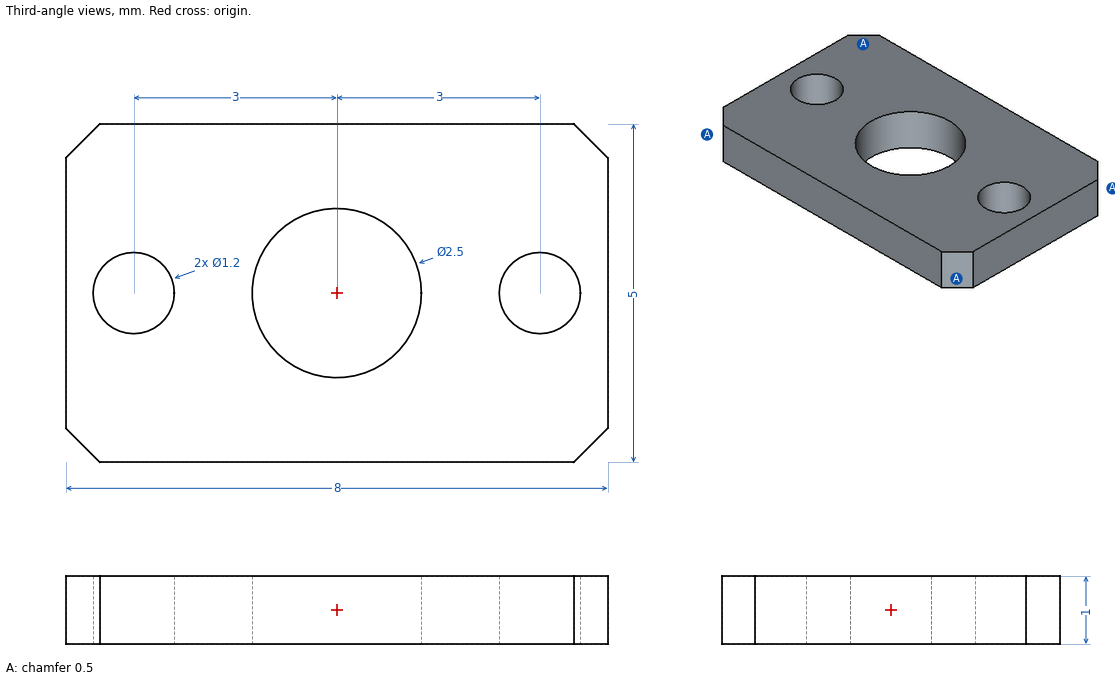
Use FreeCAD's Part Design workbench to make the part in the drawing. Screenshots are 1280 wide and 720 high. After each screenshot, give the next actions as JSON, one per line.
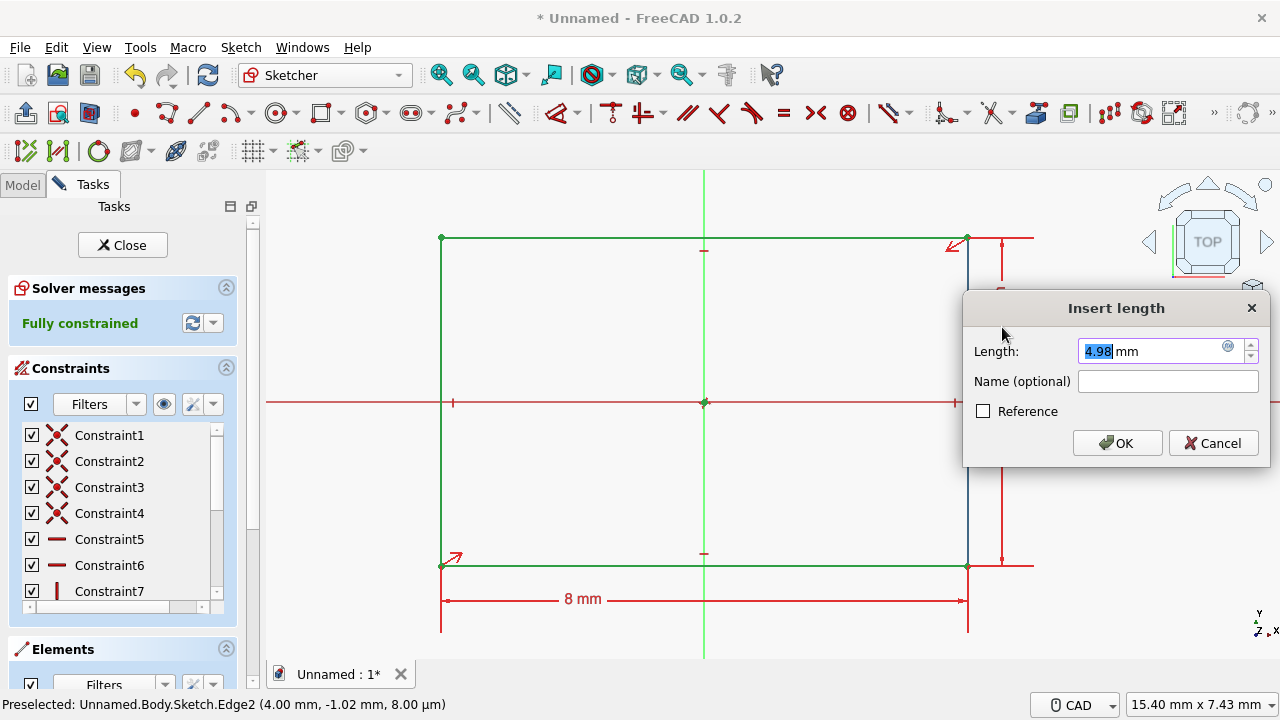
{"action": "type", "text": "5"}
{"action": "key", "text": "Return"}
{"action": "key", "text": "Escape"}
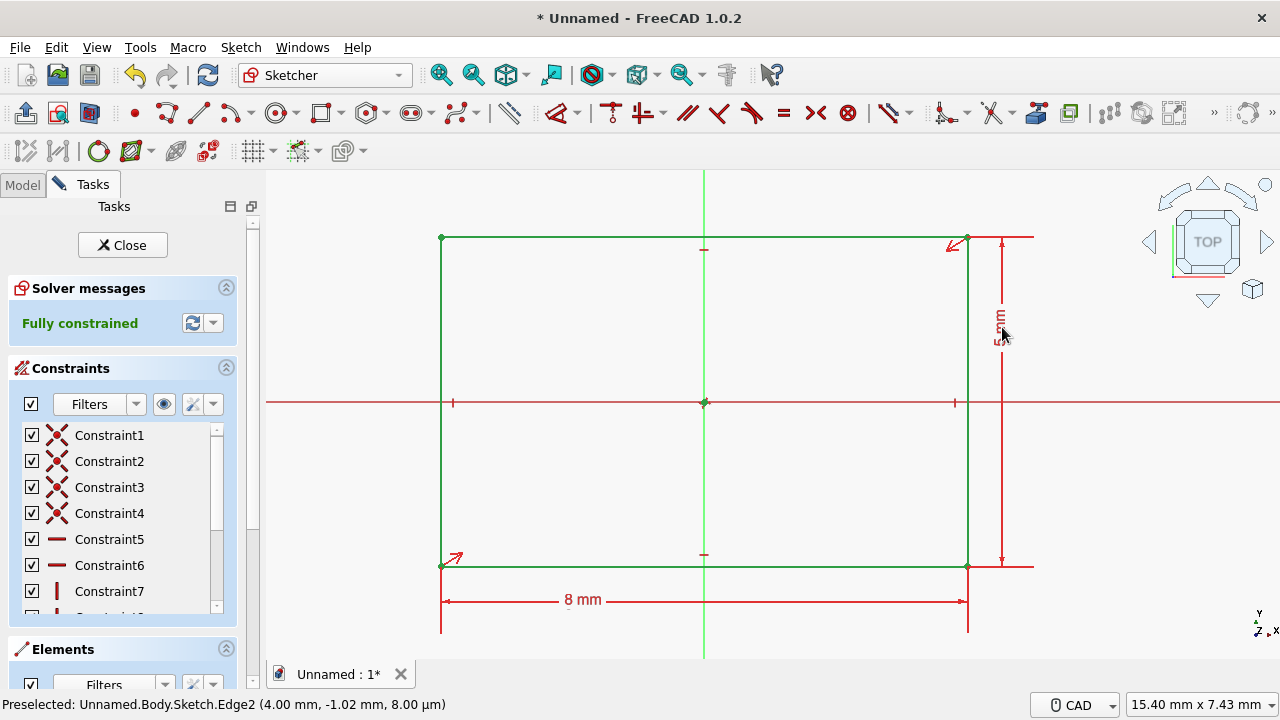
{"action": "left_click", "coordinate": [123, 245]}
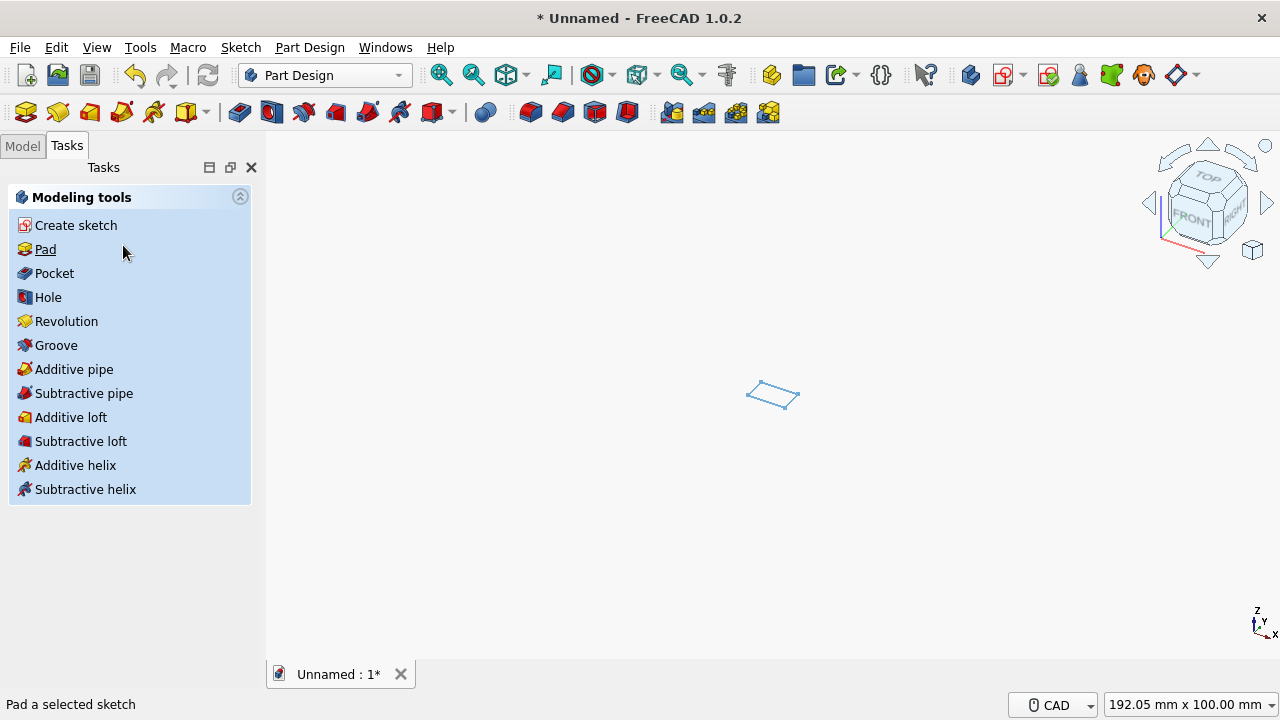
{"action": "left_click", "coordinate": [26, 112]}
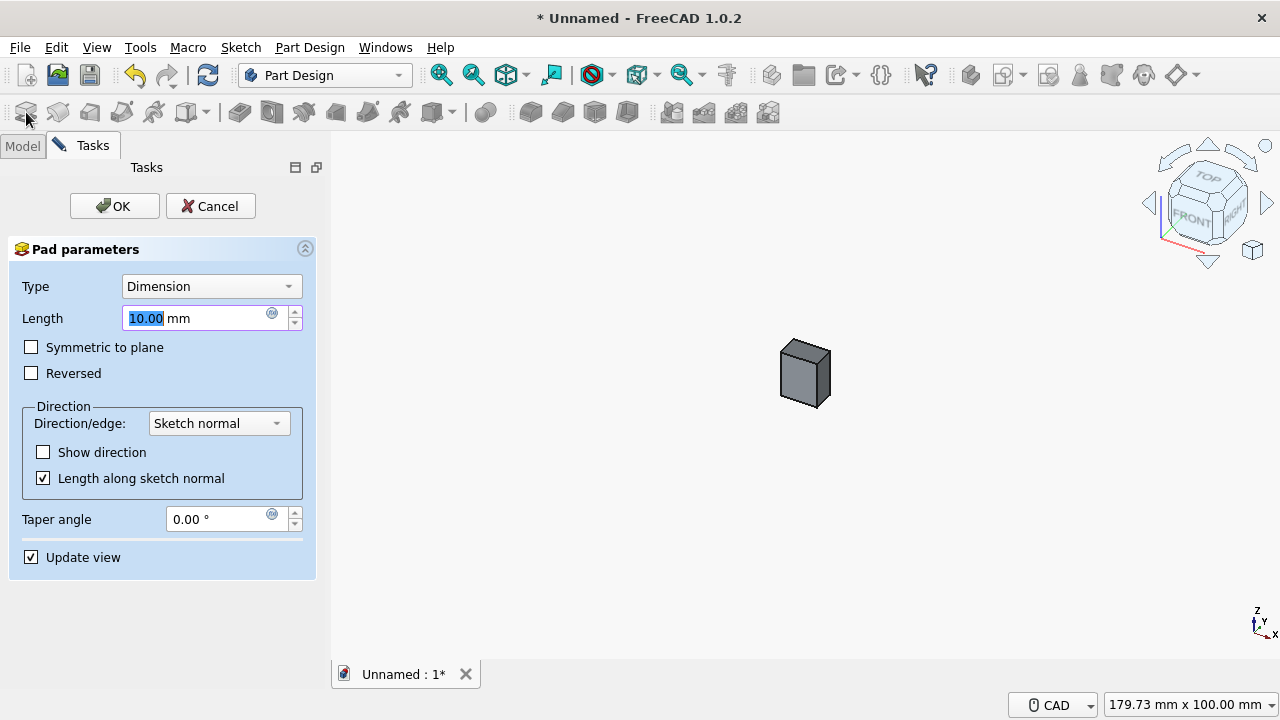
{"action": "type", "text": "1"}
{"action": "key", "text": "Tab"}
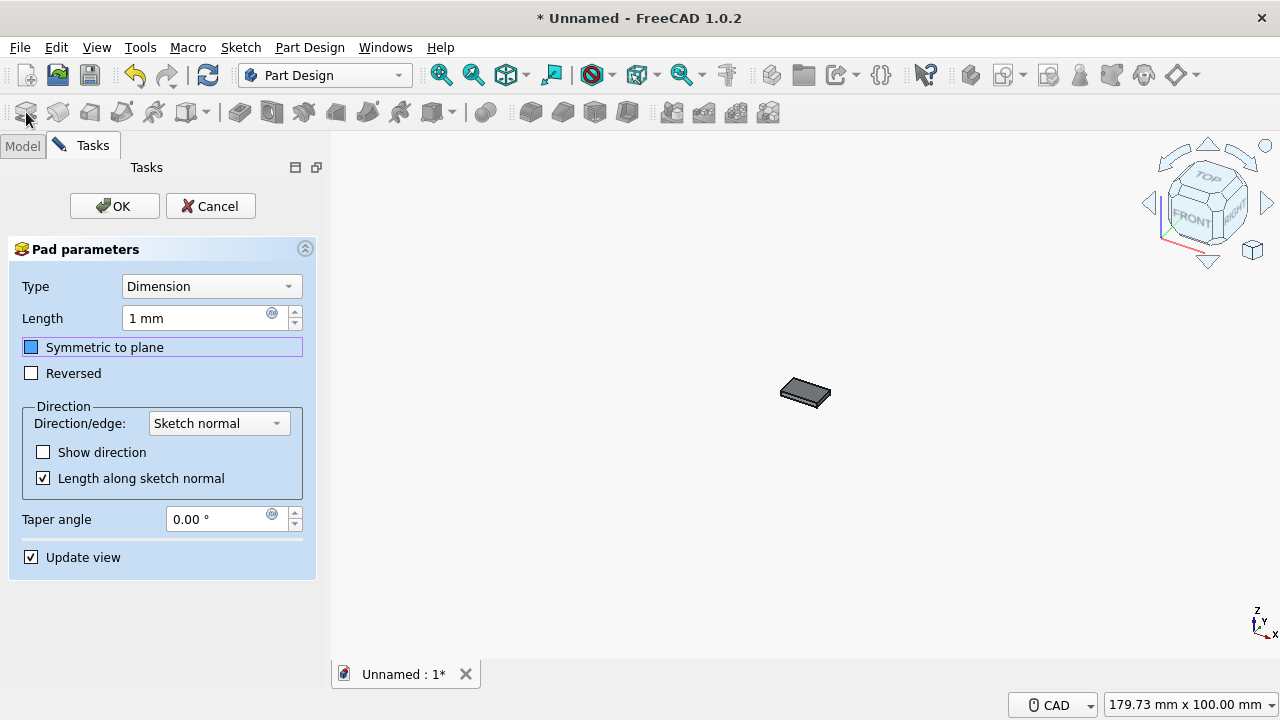
{"action": "left_click", "coordinate": [30, 347]}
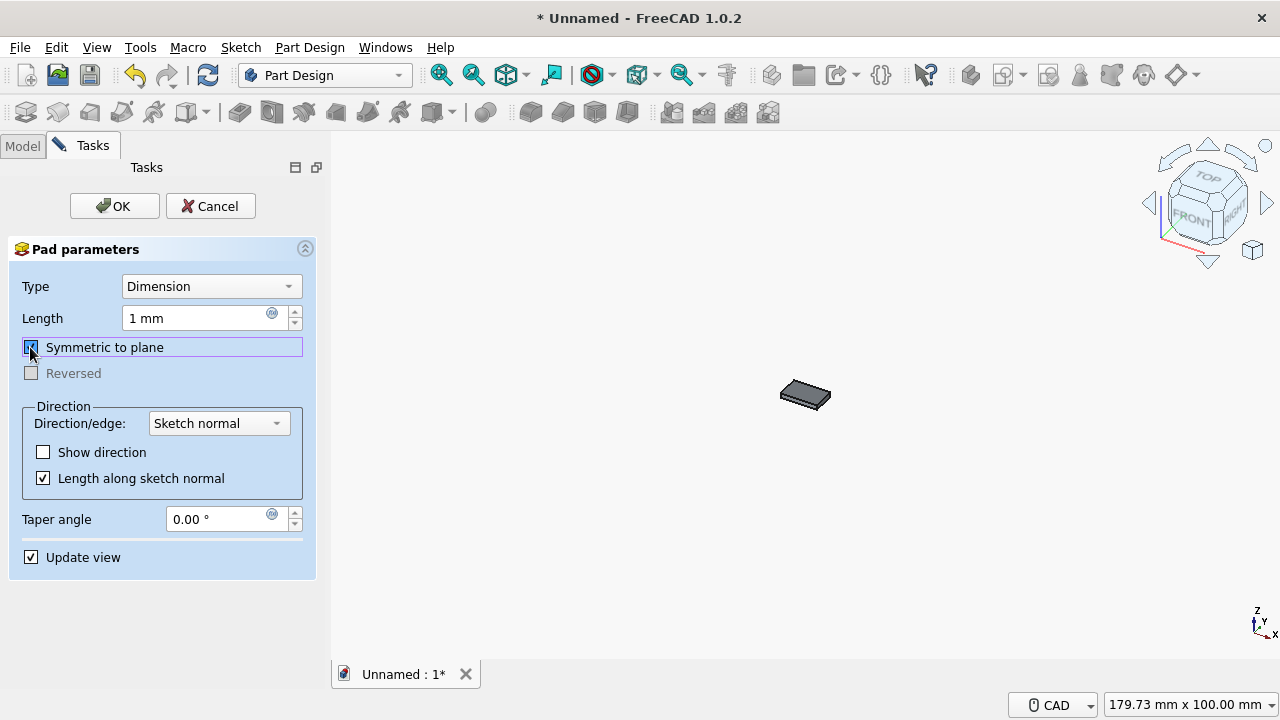
{"action": "left_click", "coordinate": [115, 206]}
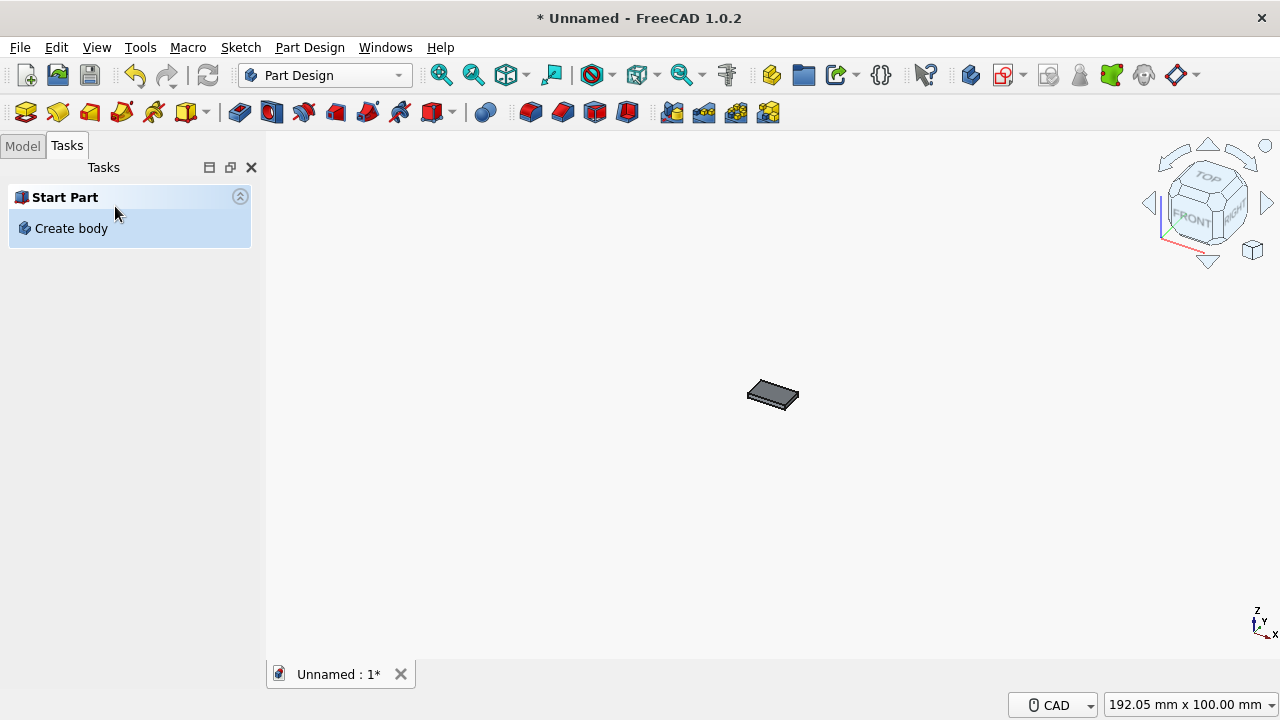
{"action": "left_click", "coordinate": [442, 76]}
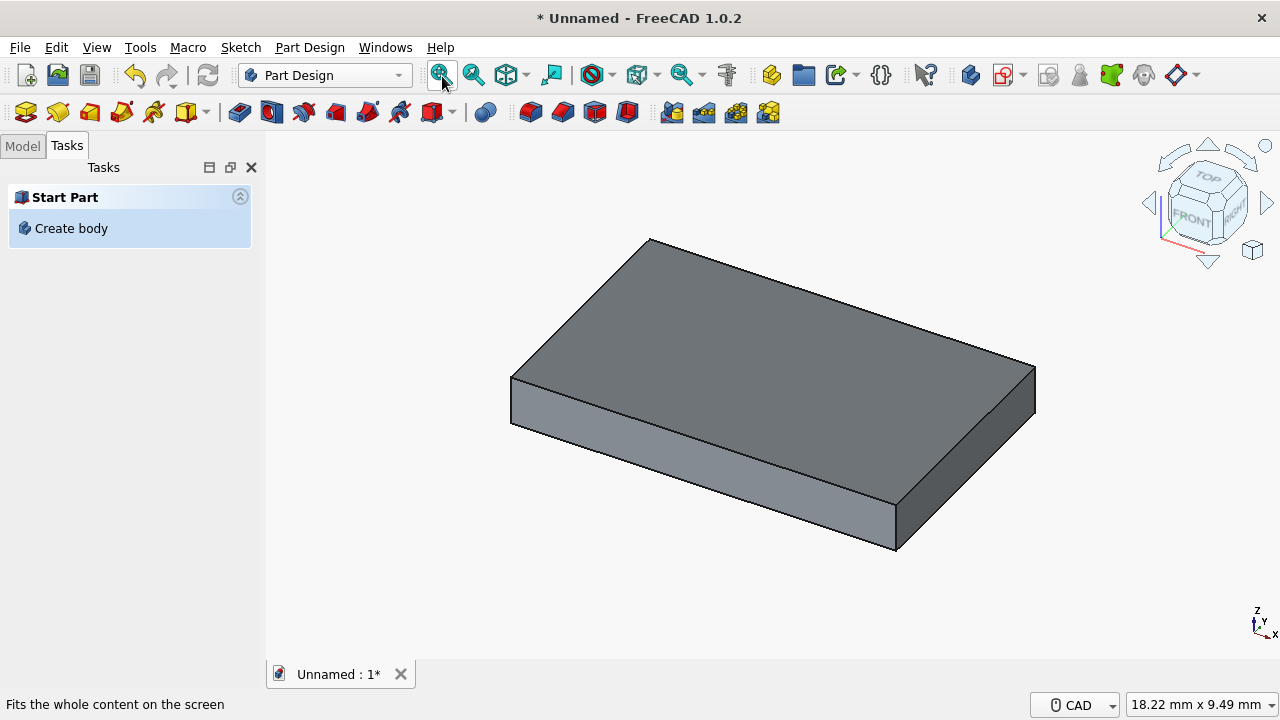
{"action": "left_click", "coordinate": [828, 389]}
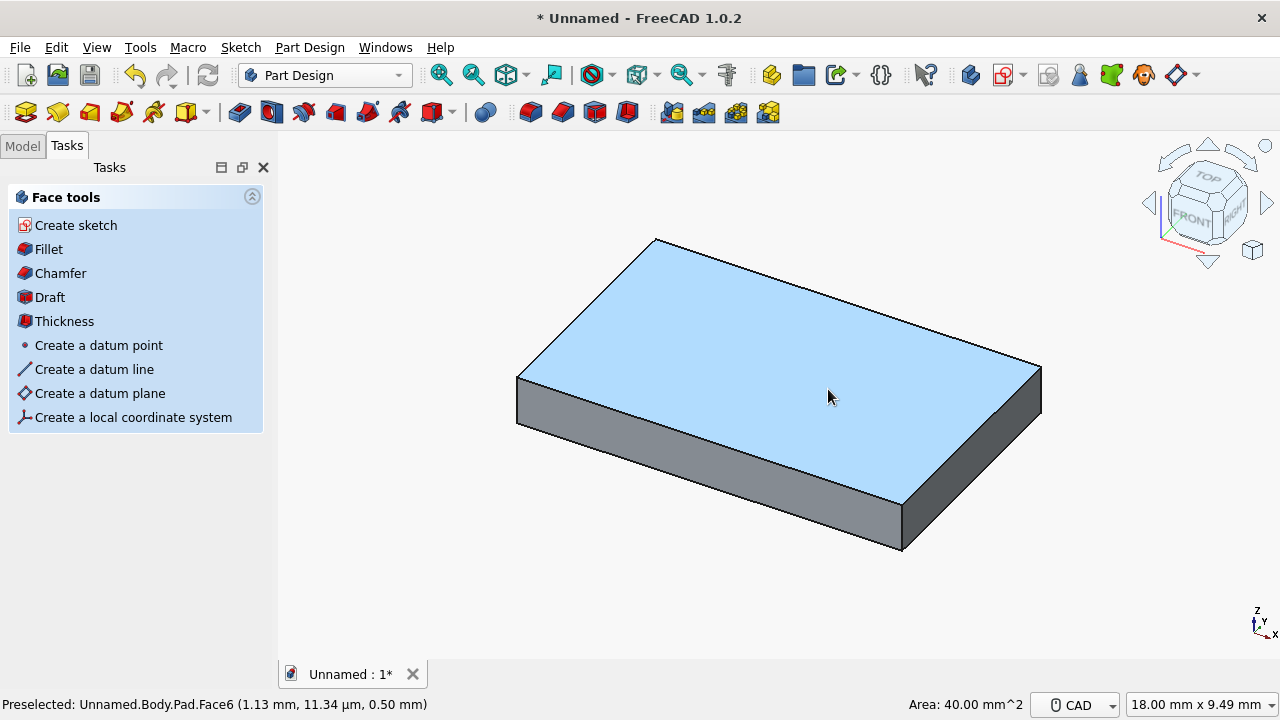
{"action": "left_click", "coordinate": [1004, 76]}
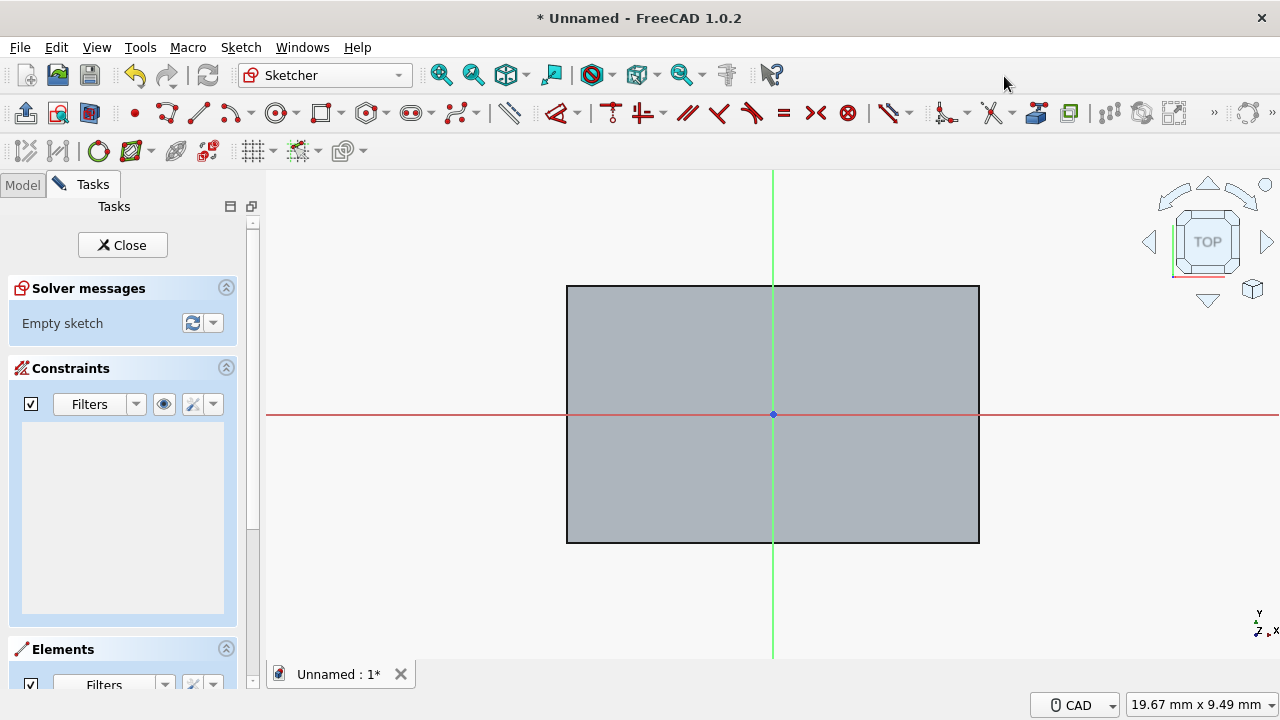
{"action": "scroll", "coordinate": [912, 414], "scroll_direction": "up", "scroll_amount": 2}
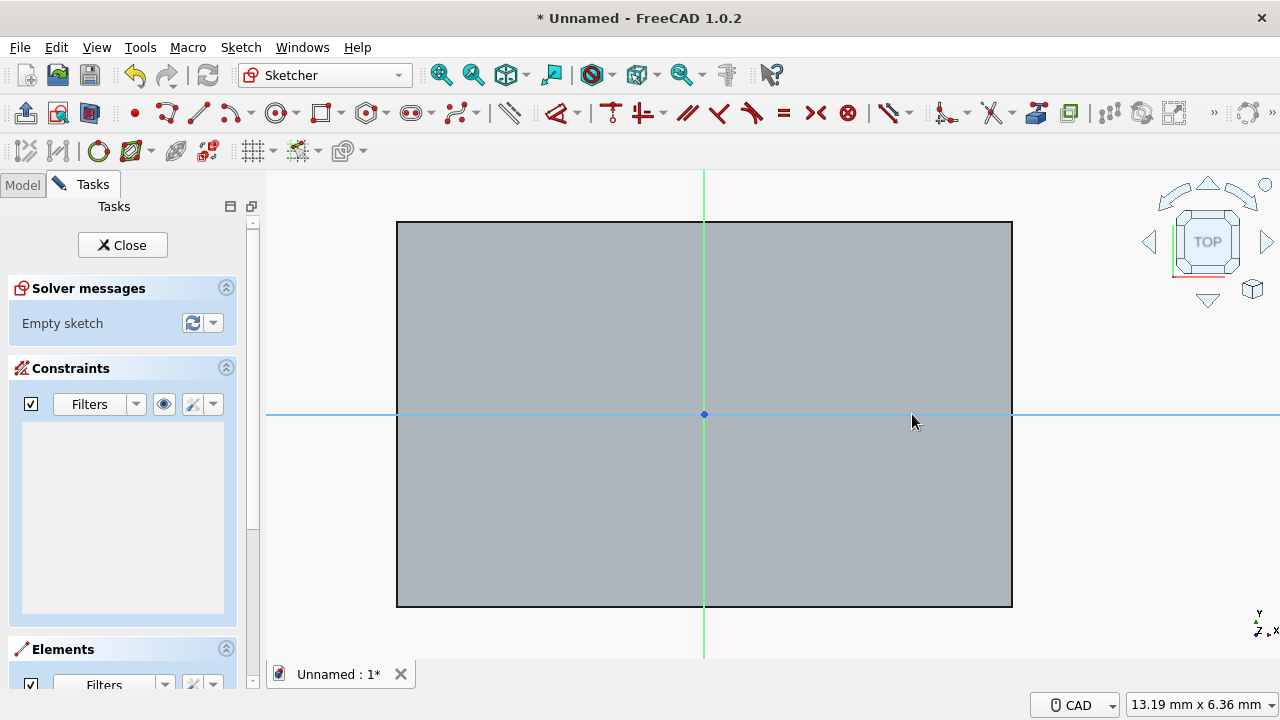
{"action": "left_click", "coordinate": [276, 114]}